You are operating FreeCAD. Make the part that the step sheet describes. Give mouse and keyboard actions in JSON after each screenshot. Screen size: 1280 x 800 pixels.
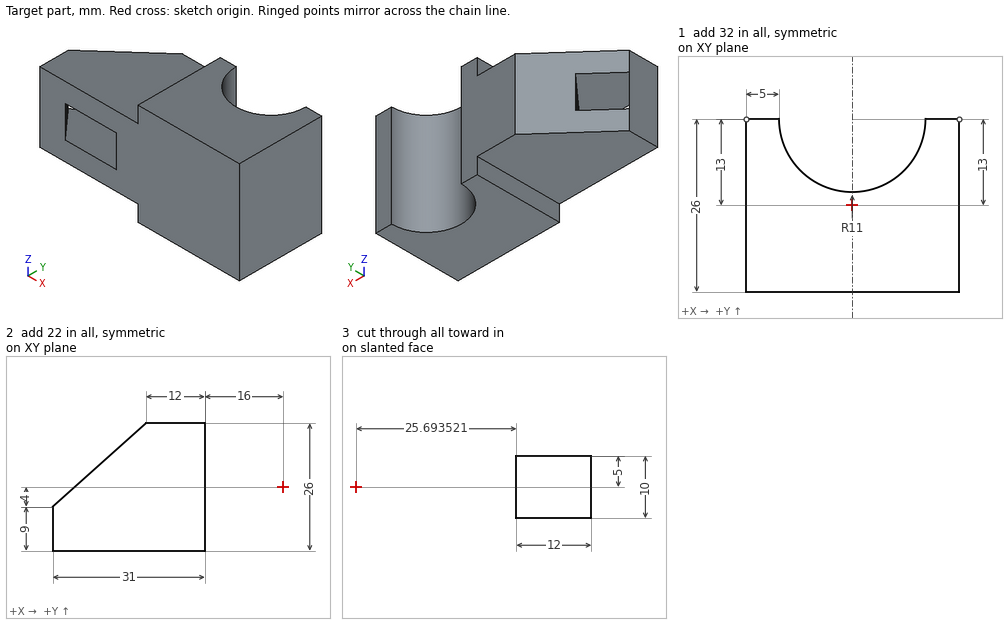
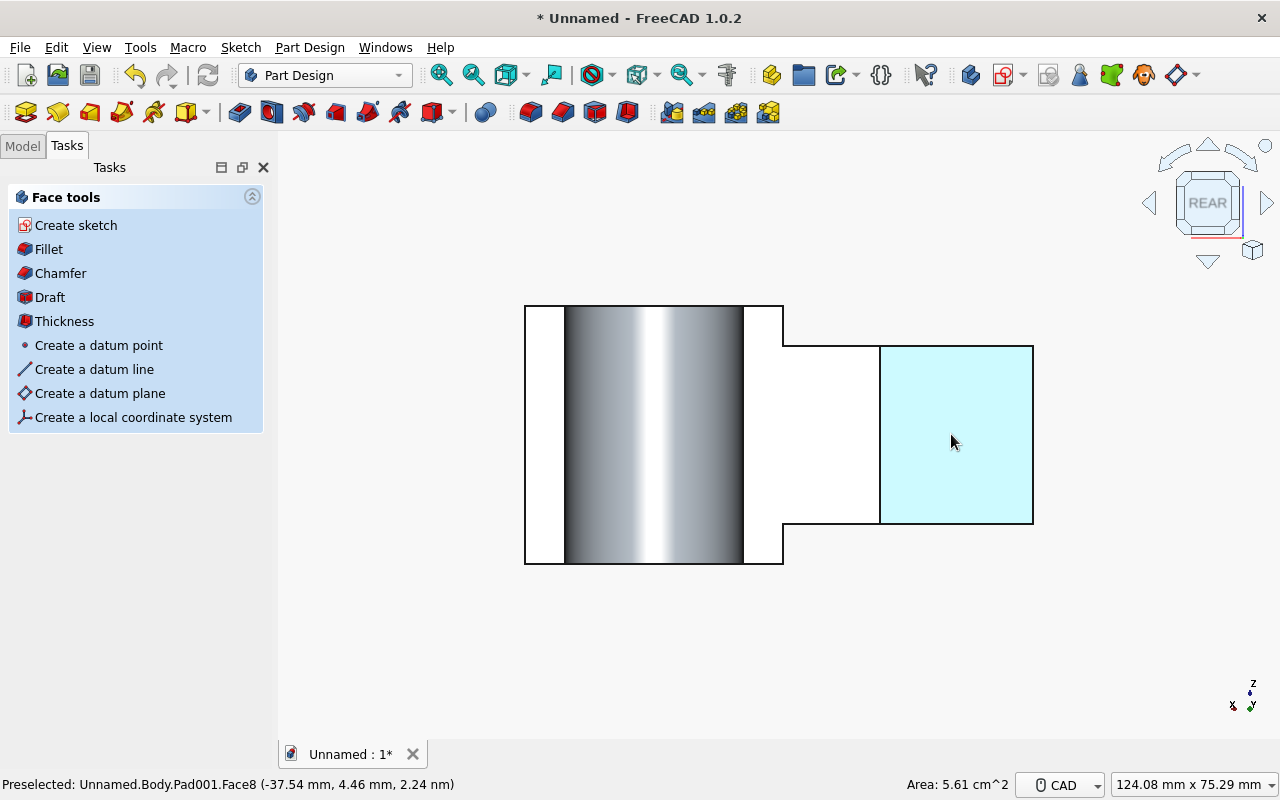
{"action": "left_click", "coordinate": [1004, 76]}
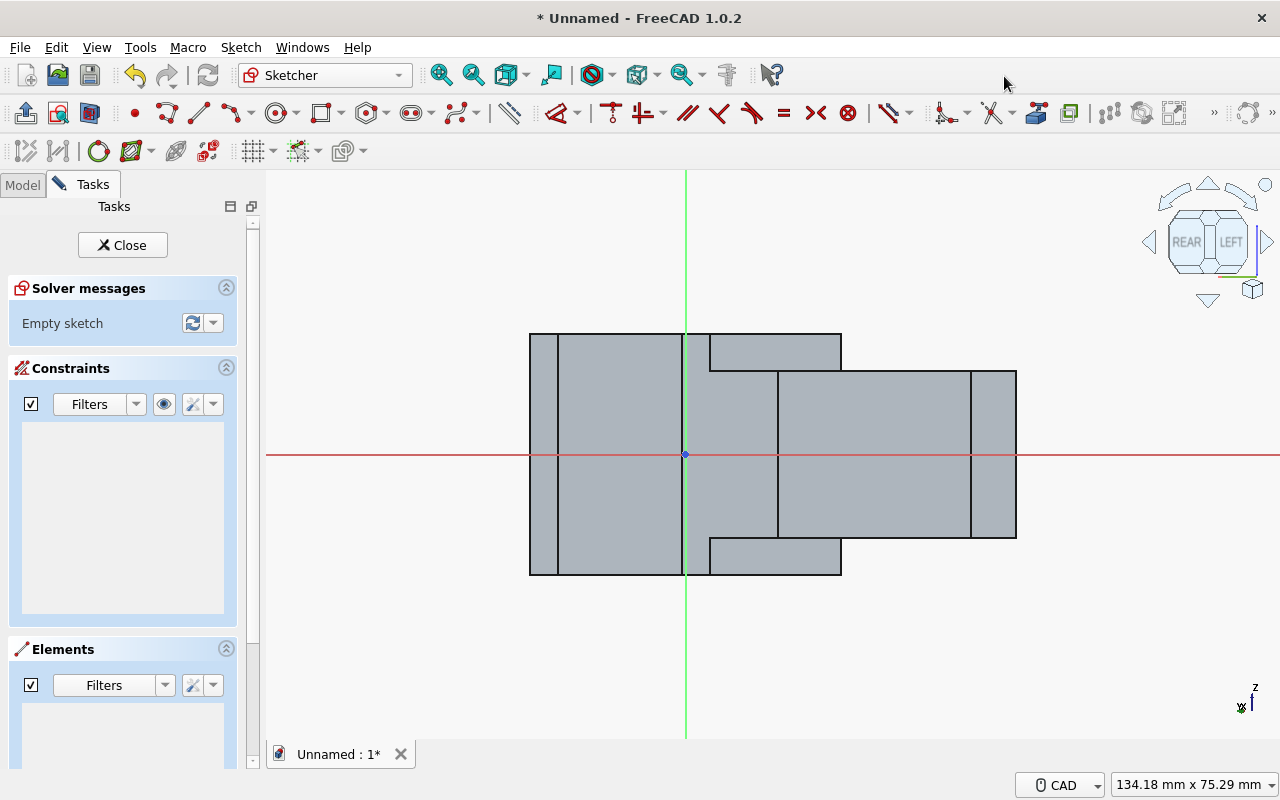
{"action": "key", "text": "q s"}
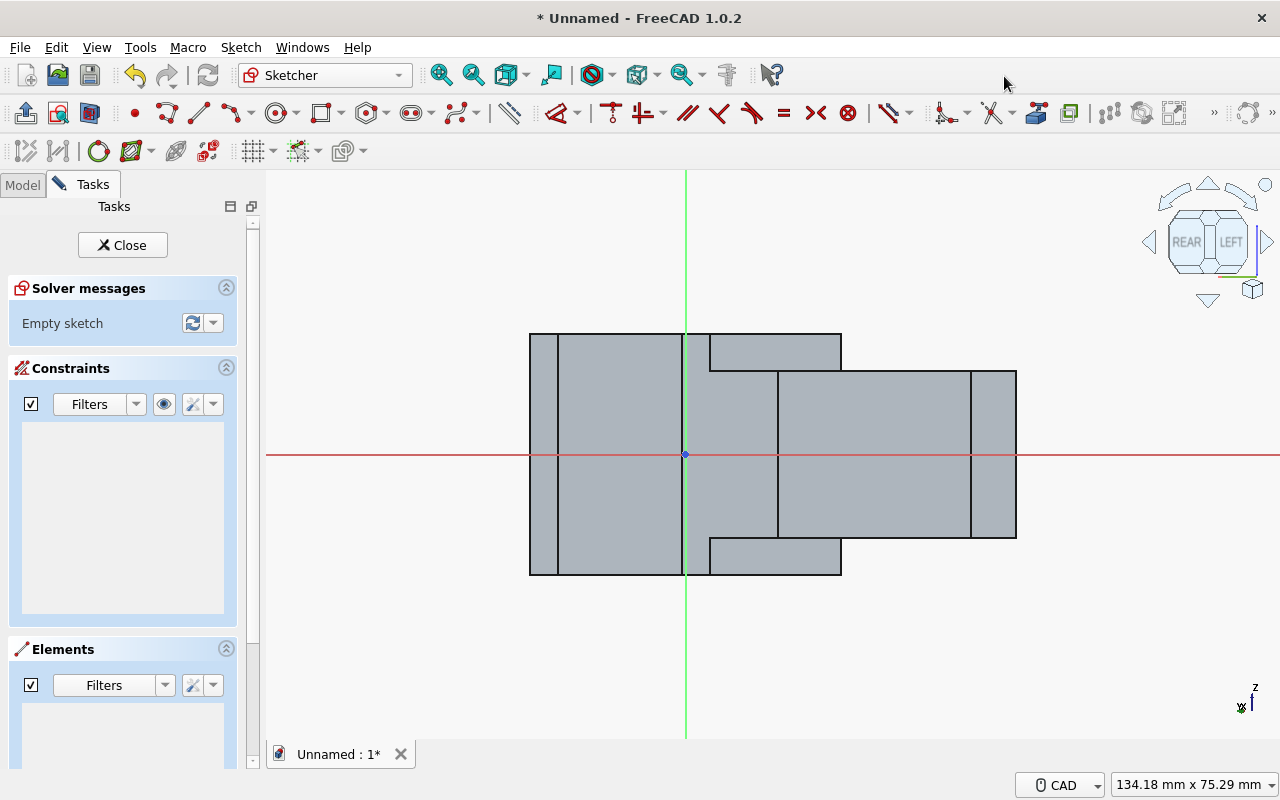
{"action": "scroll", "coordinate": [981, 454], "scroll_direction": "up", "scroll_amount": 8}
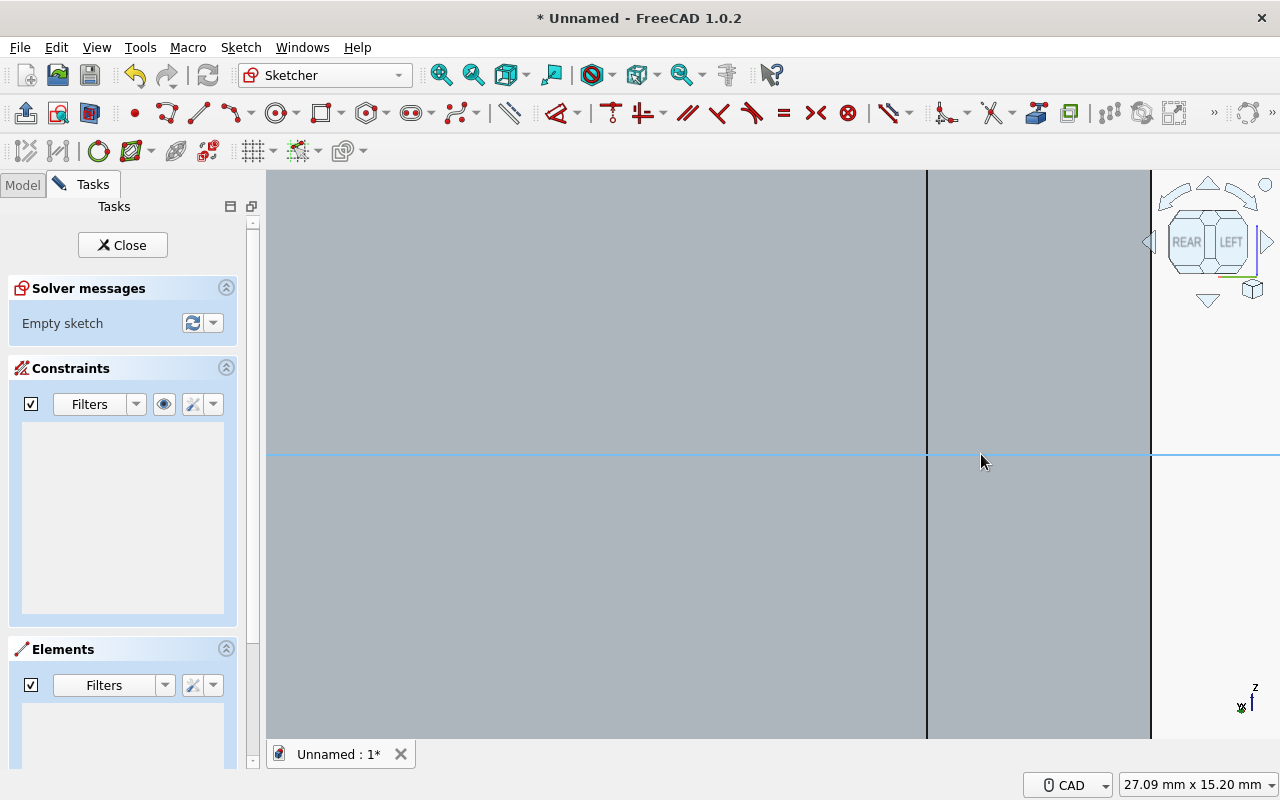
{"action": "key", "text": "g r"}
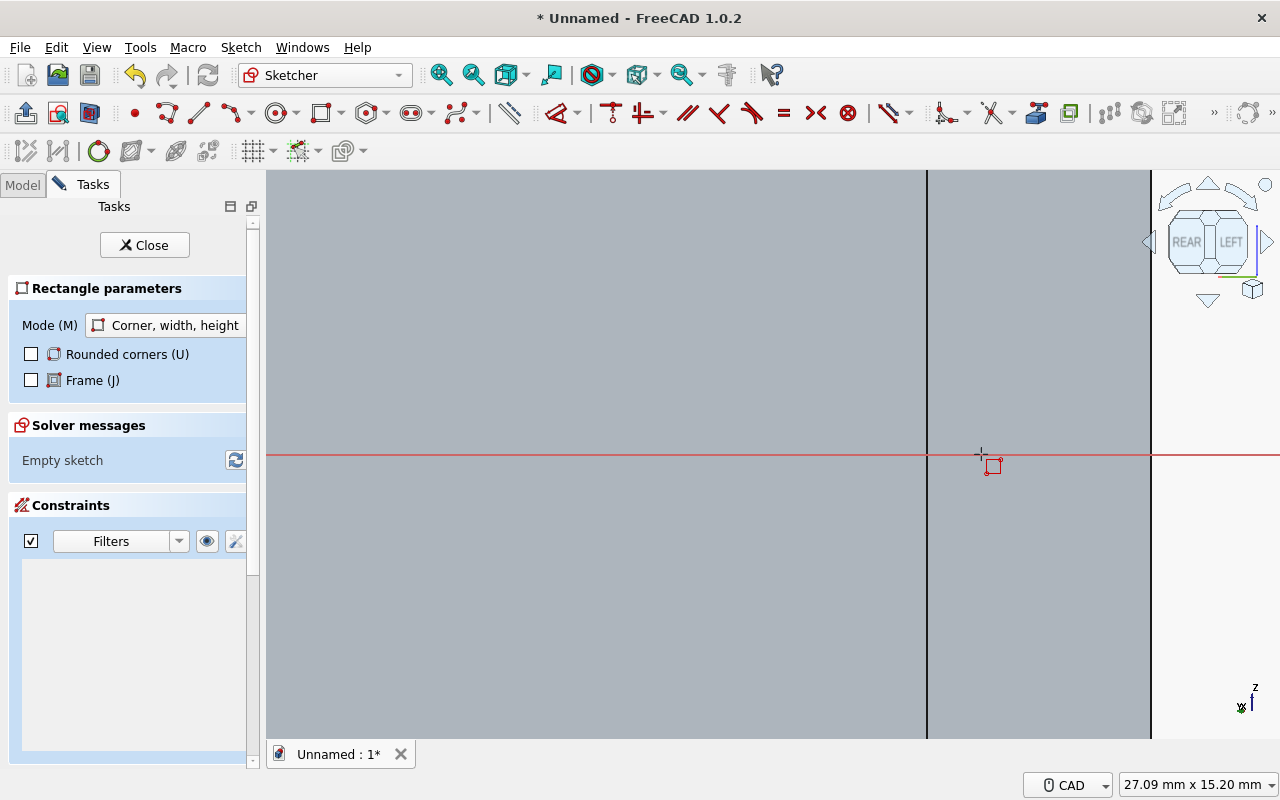
{"action": "left_click", "coordinate": [477, 267]}
{"action": "mouse_move", "coordinate": [927, 642]}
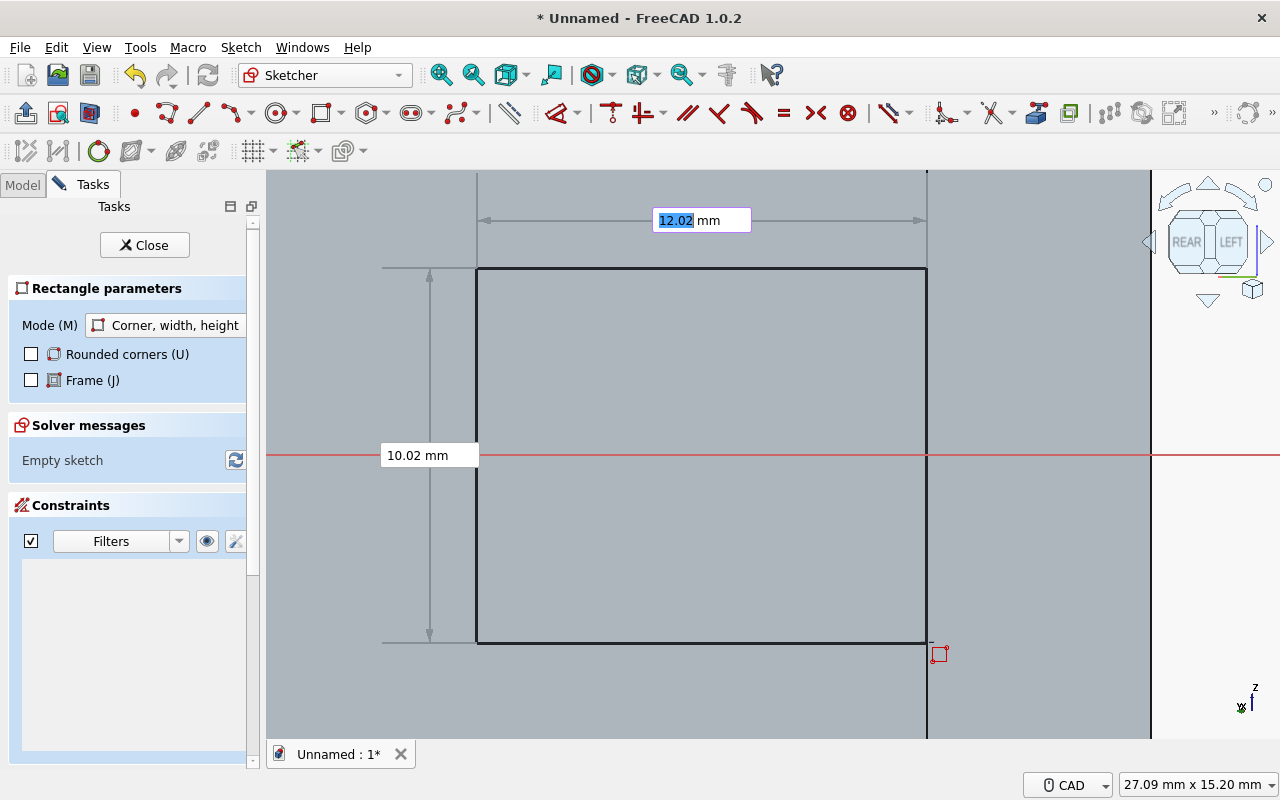
{"action": "type", "text": "12"}
{"action": "key", "text": "Tab"}
{"action": "type", "text": "10"}
{"action": "key", "text": "Return"}
{"action": "key", "text": "Escape"}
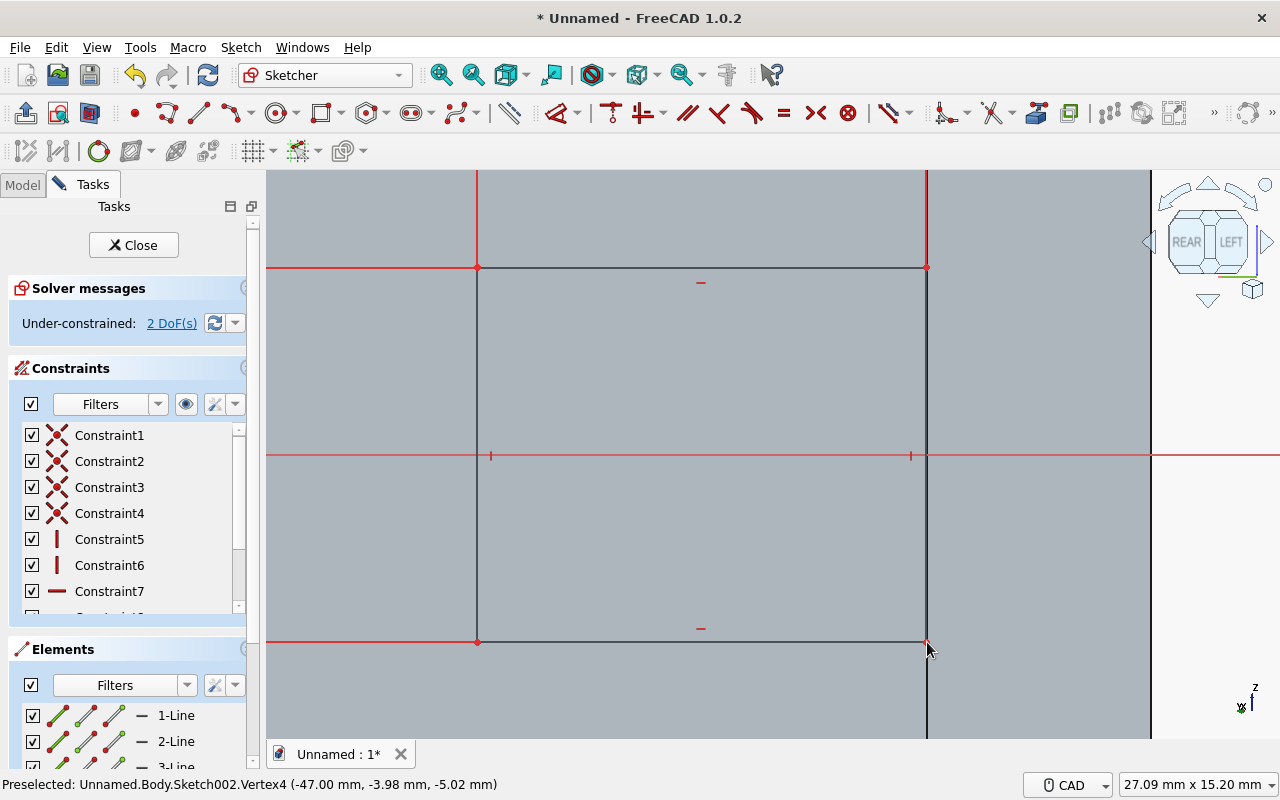
{"action": "key", "text": "d"}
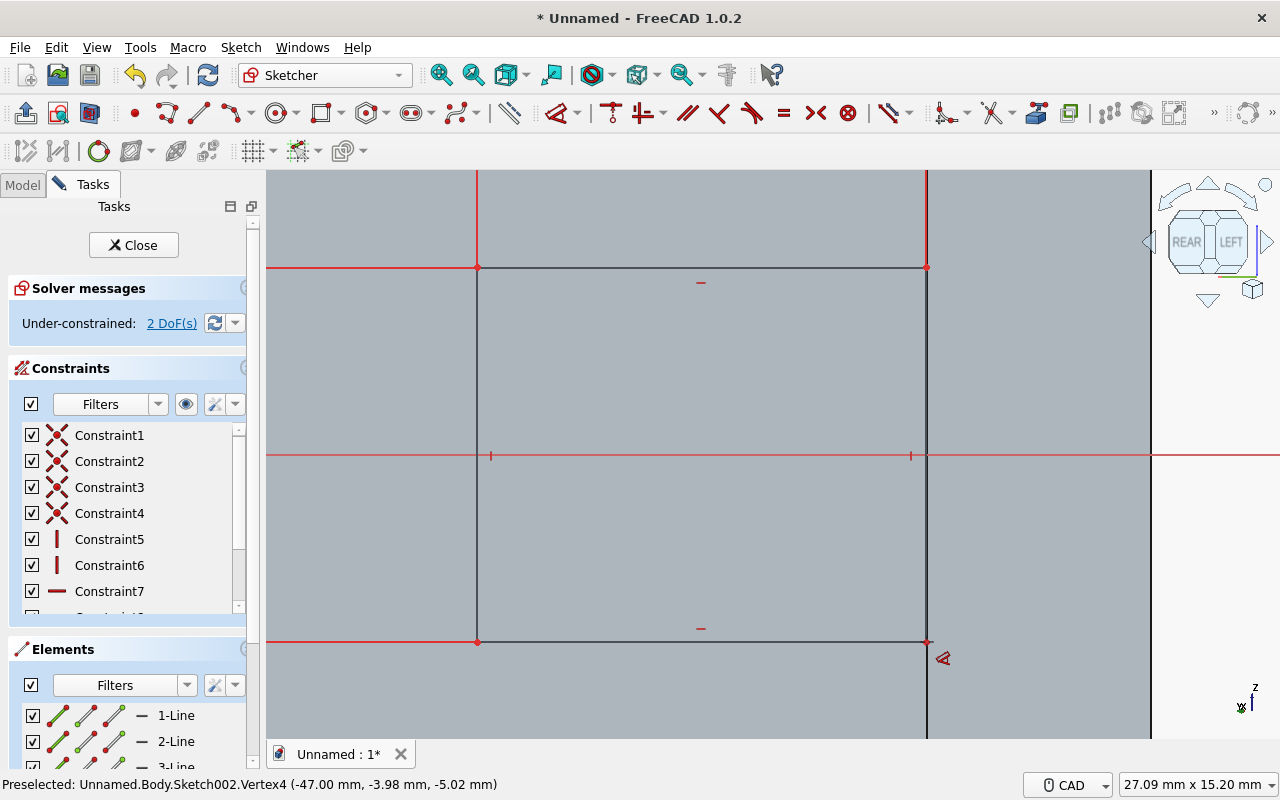
{"action": "left_click", "coordinate": [477, 268]}
{"action": "left_click", "coordinate": [511, 361]}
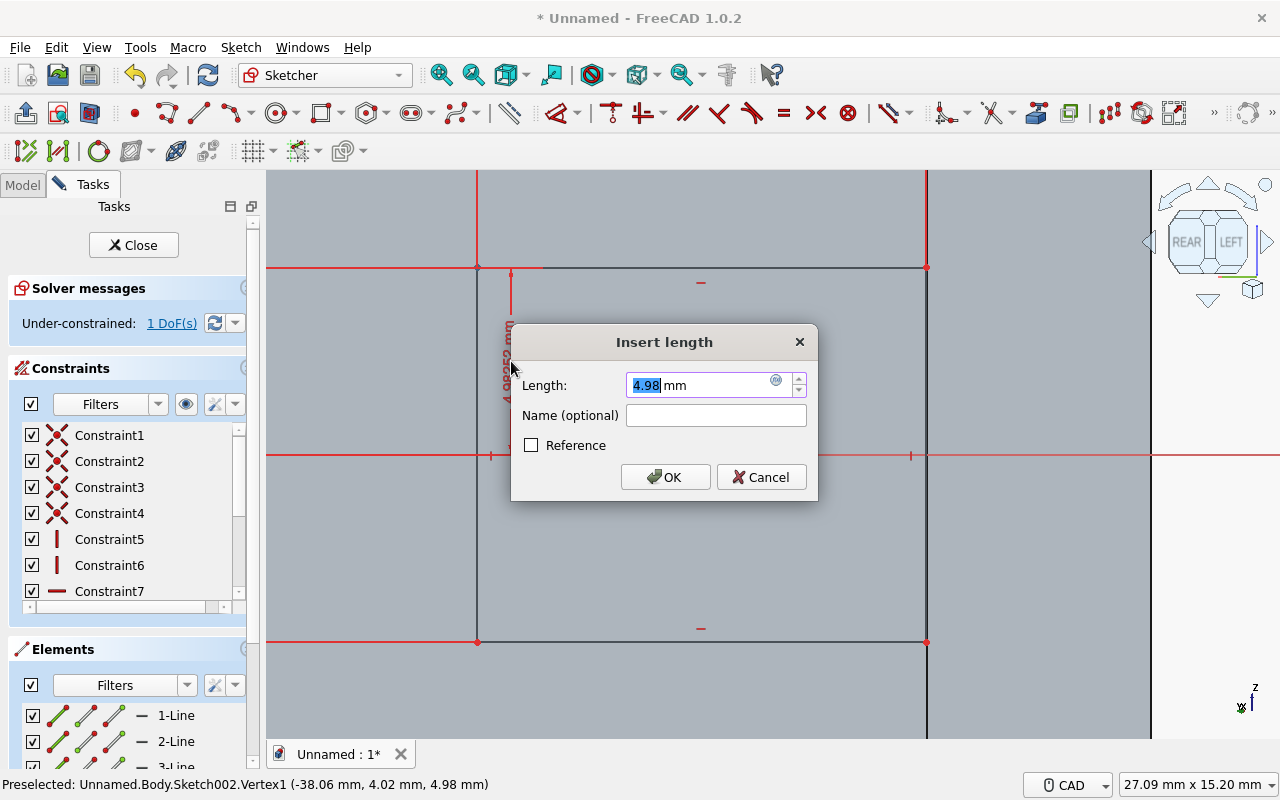
{"action": "type", "text": "5"}
{"action": "key", "text": "Return"}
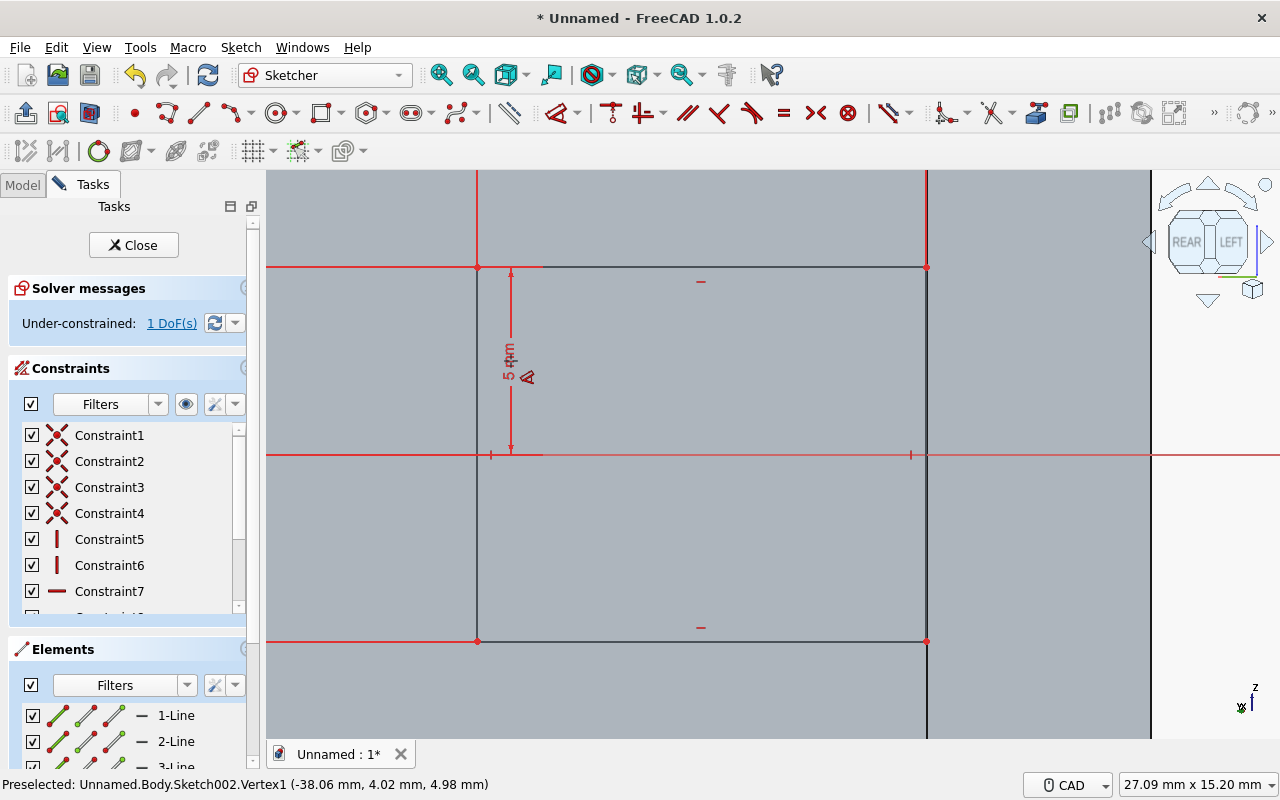
{"action": "left_click", "coordinate": [477, 267]}
{"action": "left_click", "coordinate": [386, 233]}